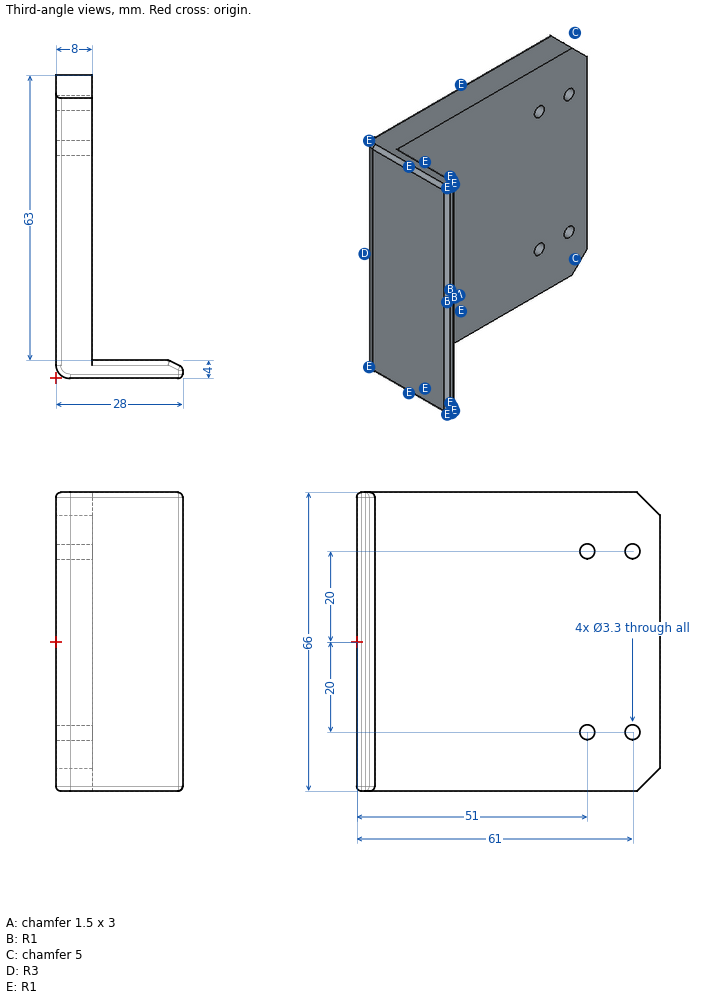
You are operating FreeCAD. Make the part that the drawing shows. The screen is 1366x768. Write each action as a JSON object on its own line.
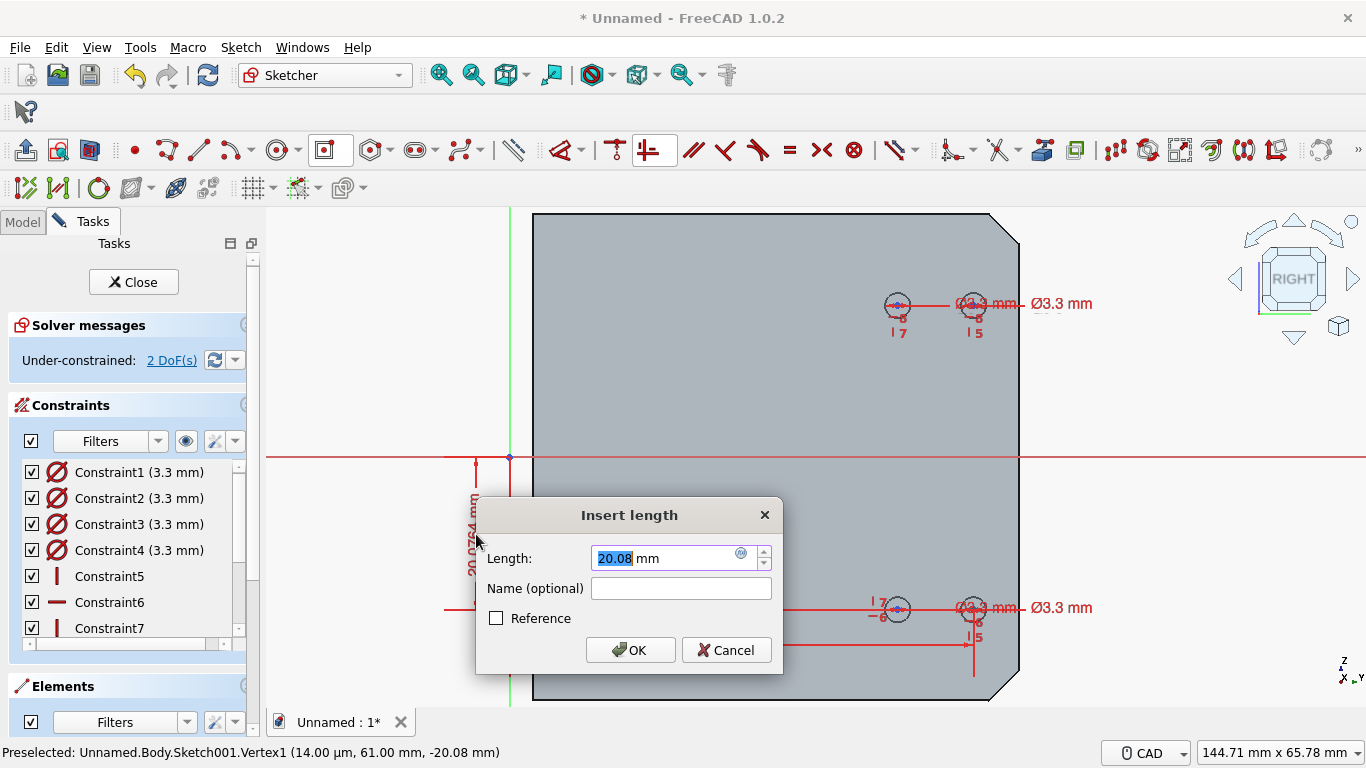
{"action": "type", "text": "20"}
{"action": "key", "text": "Return"}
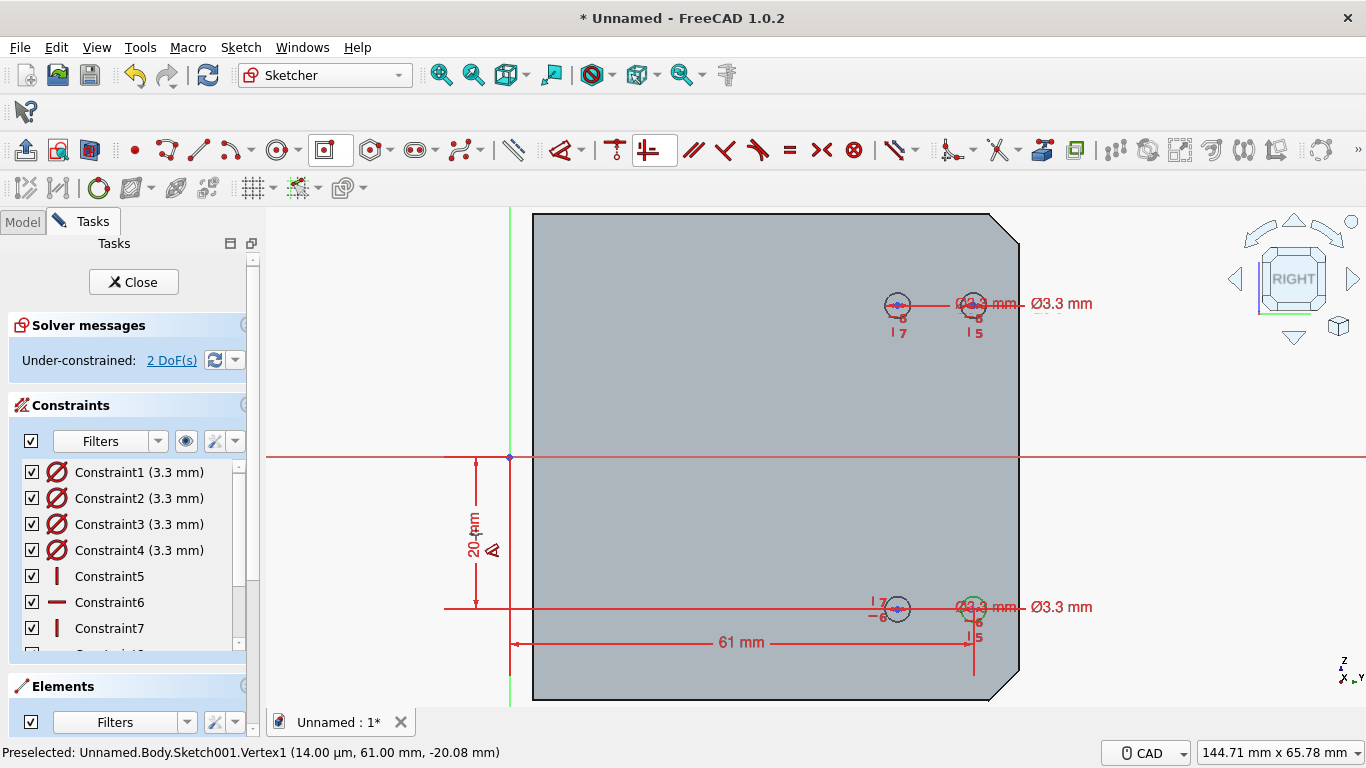
{"action": "left_click", "coordinate": [974, 306]}
{"action": "left_click", "coordinate": [476, 381]}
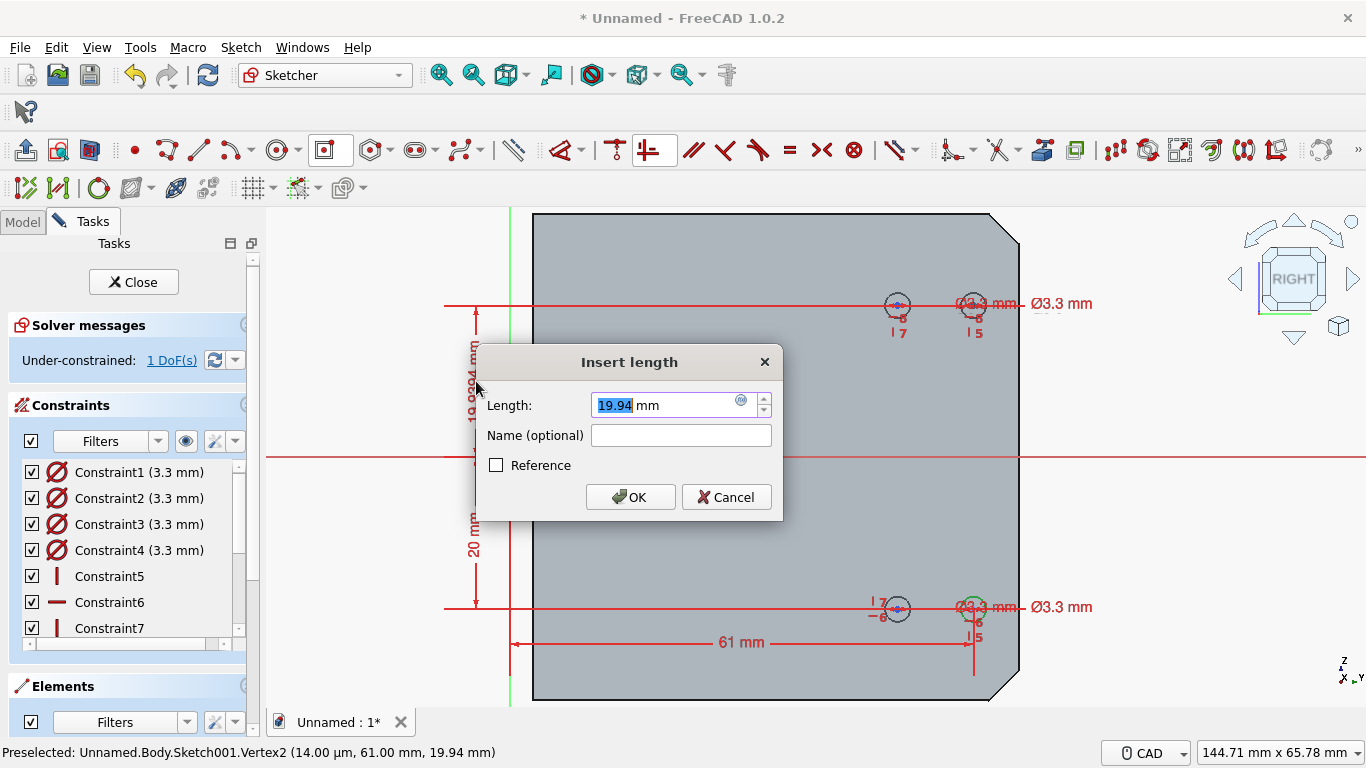
{"action": "type", "text": "20"}
{"action": "key", "text": "Return"}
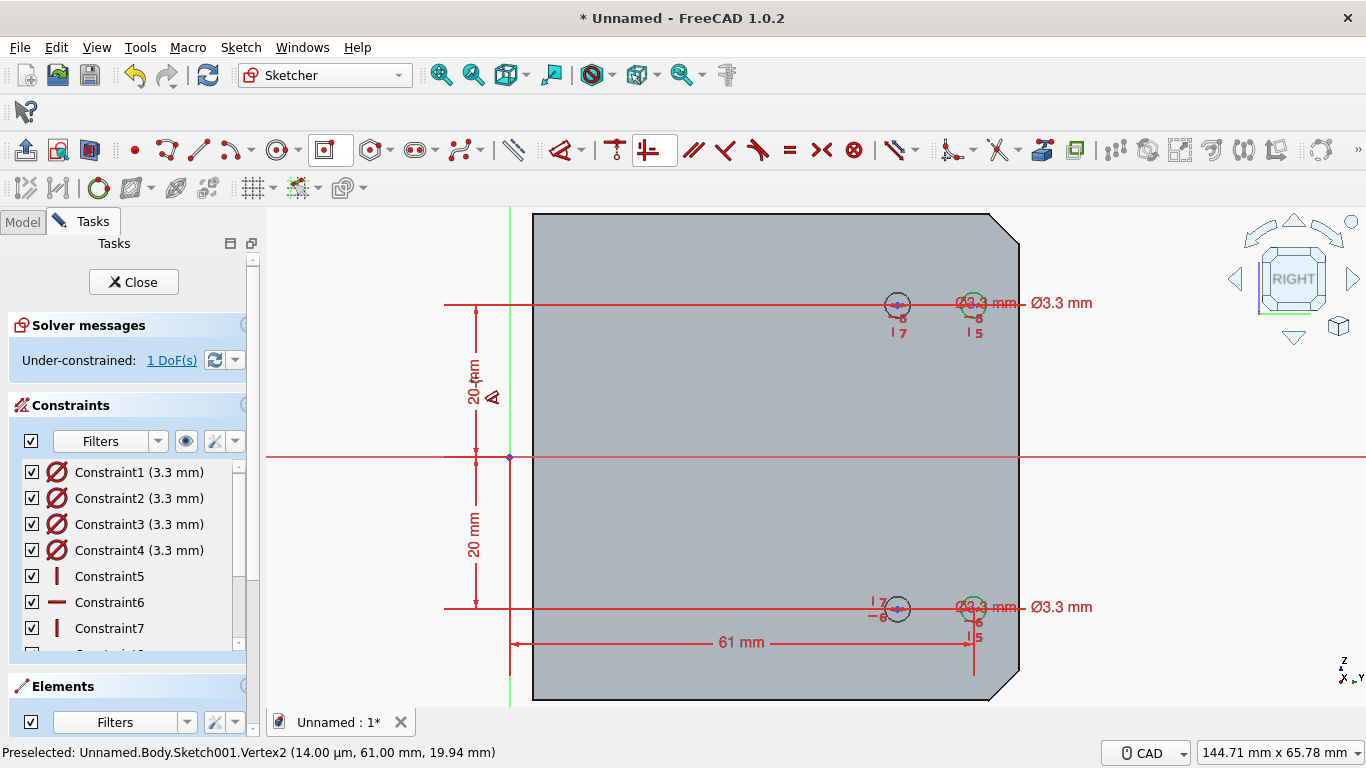
{"action": "left_click", "coordinate": [898, 609]}
{"action": "left_click", "coordinate": [615, 643]}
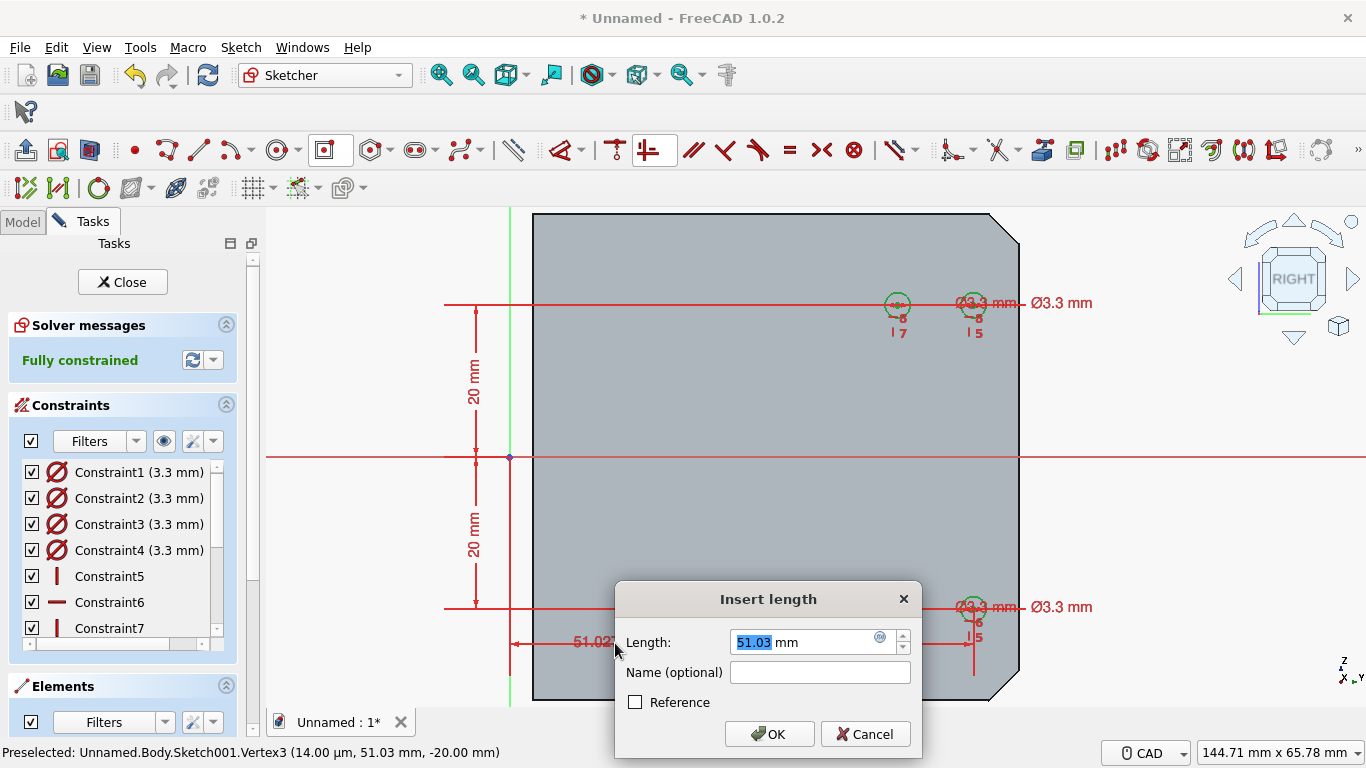
{"action": "type", "text": "51"}
{"action": "key", "text": "Return"}
{"action": "key", "text": "Escape"}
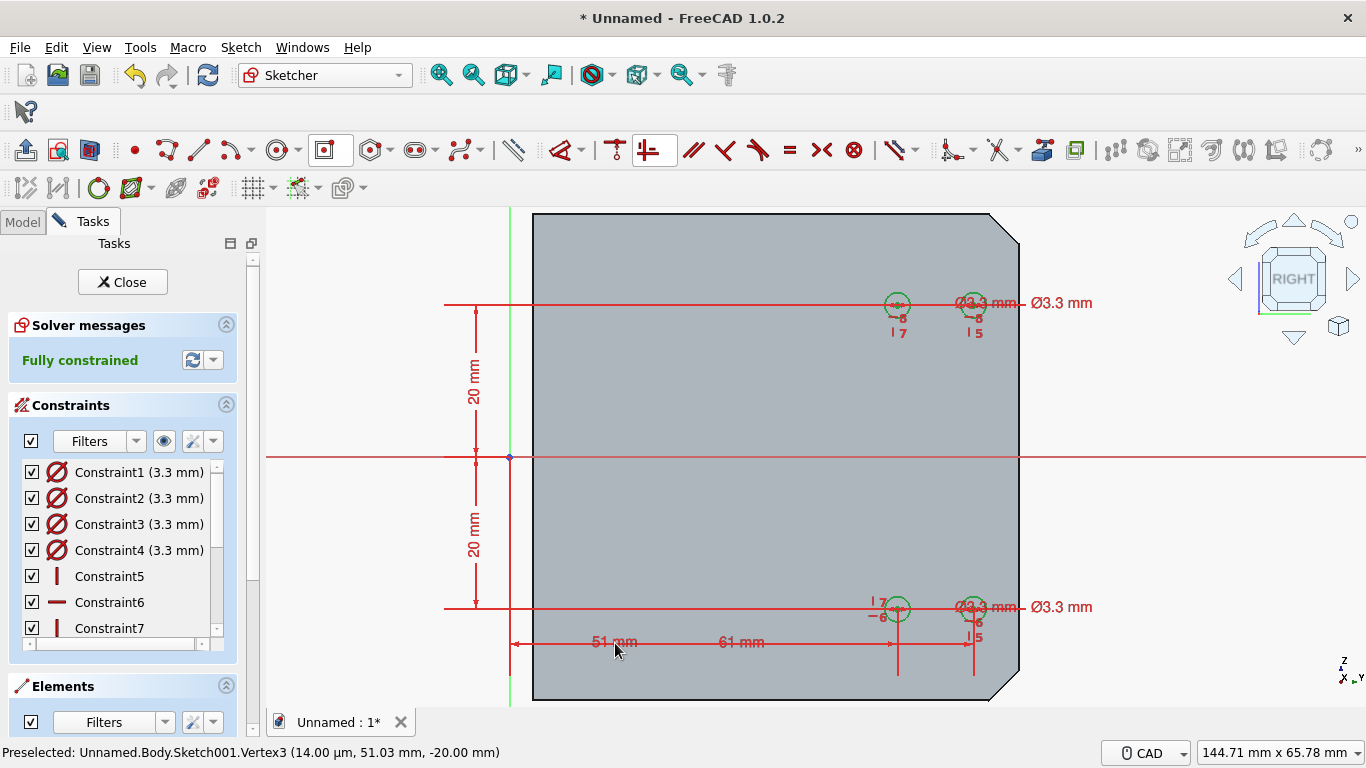
{"action": "left_click", "coordinate": [123, 282]}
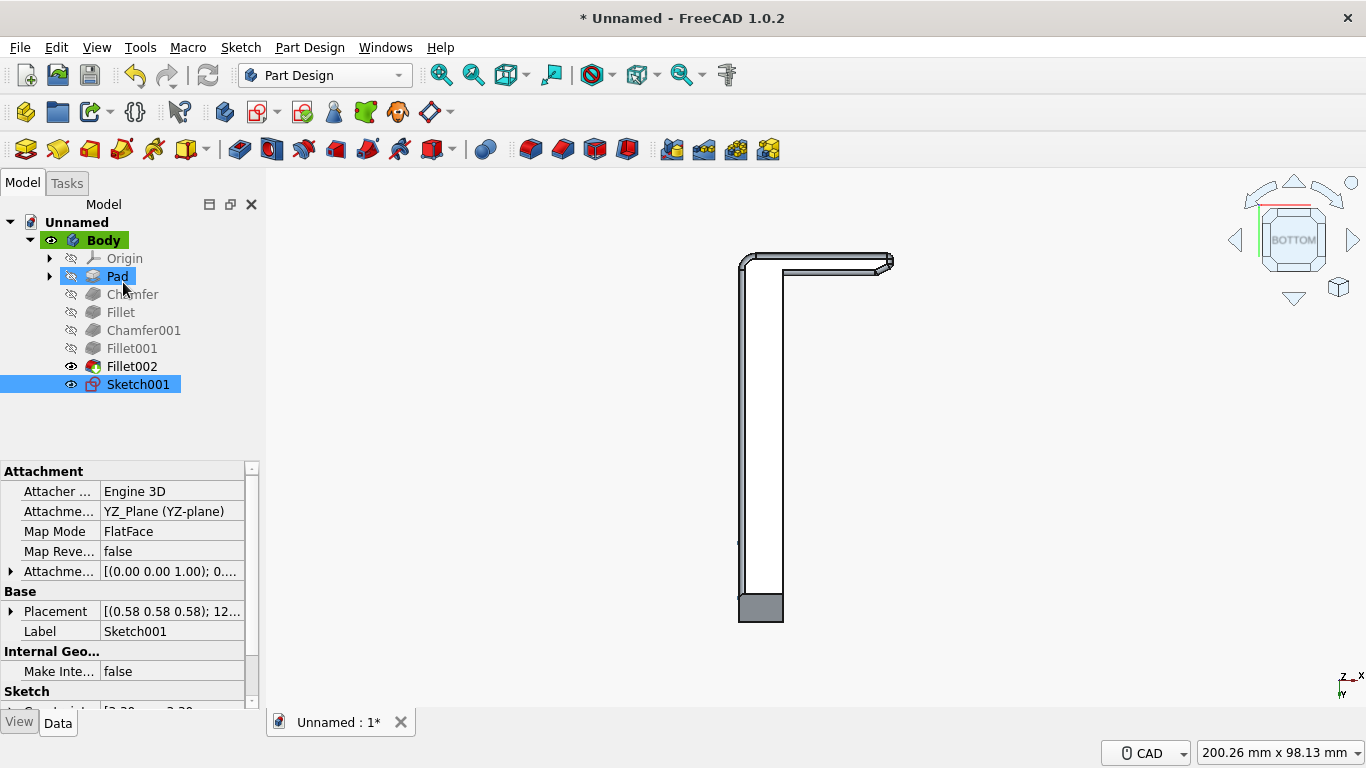
{"action": "left_click", "coordinate": [272, 150]}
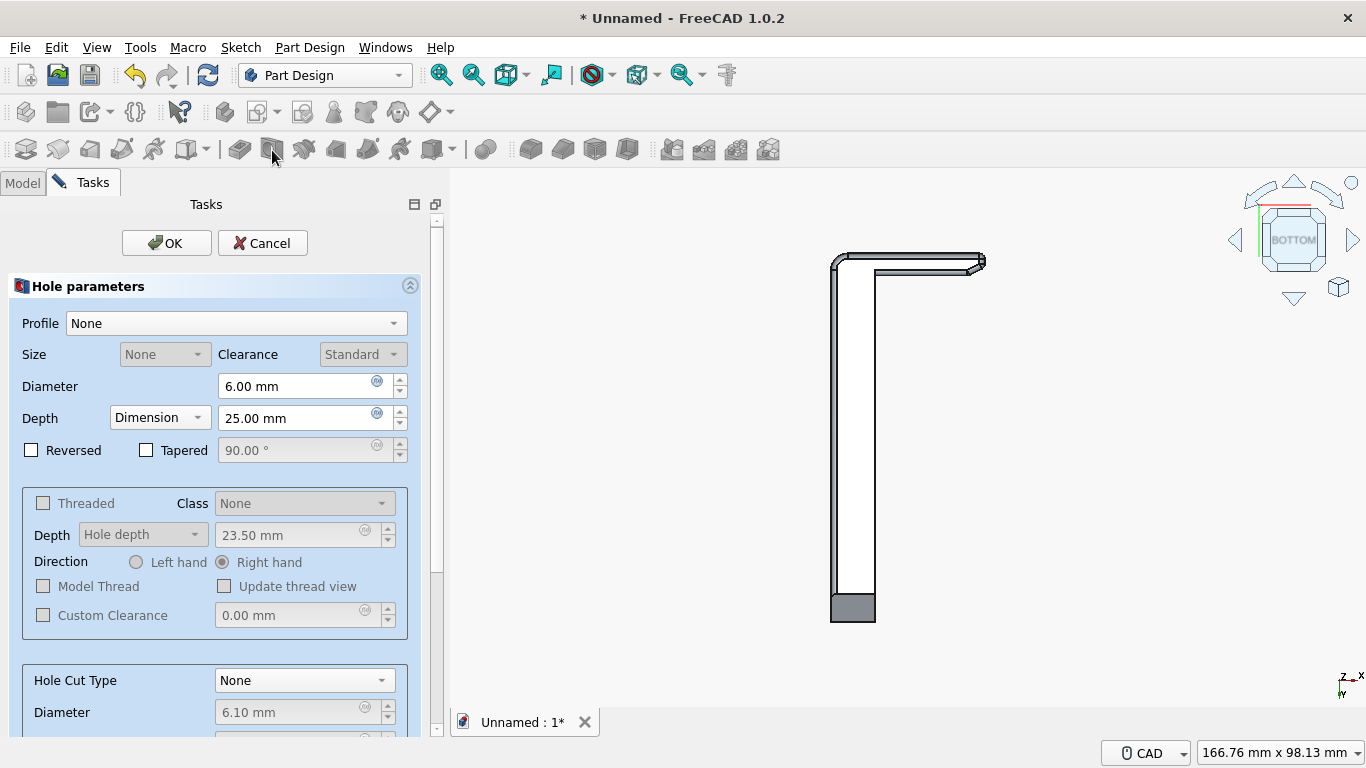
{"action": "triple_click", "coordinate": [305, 386]}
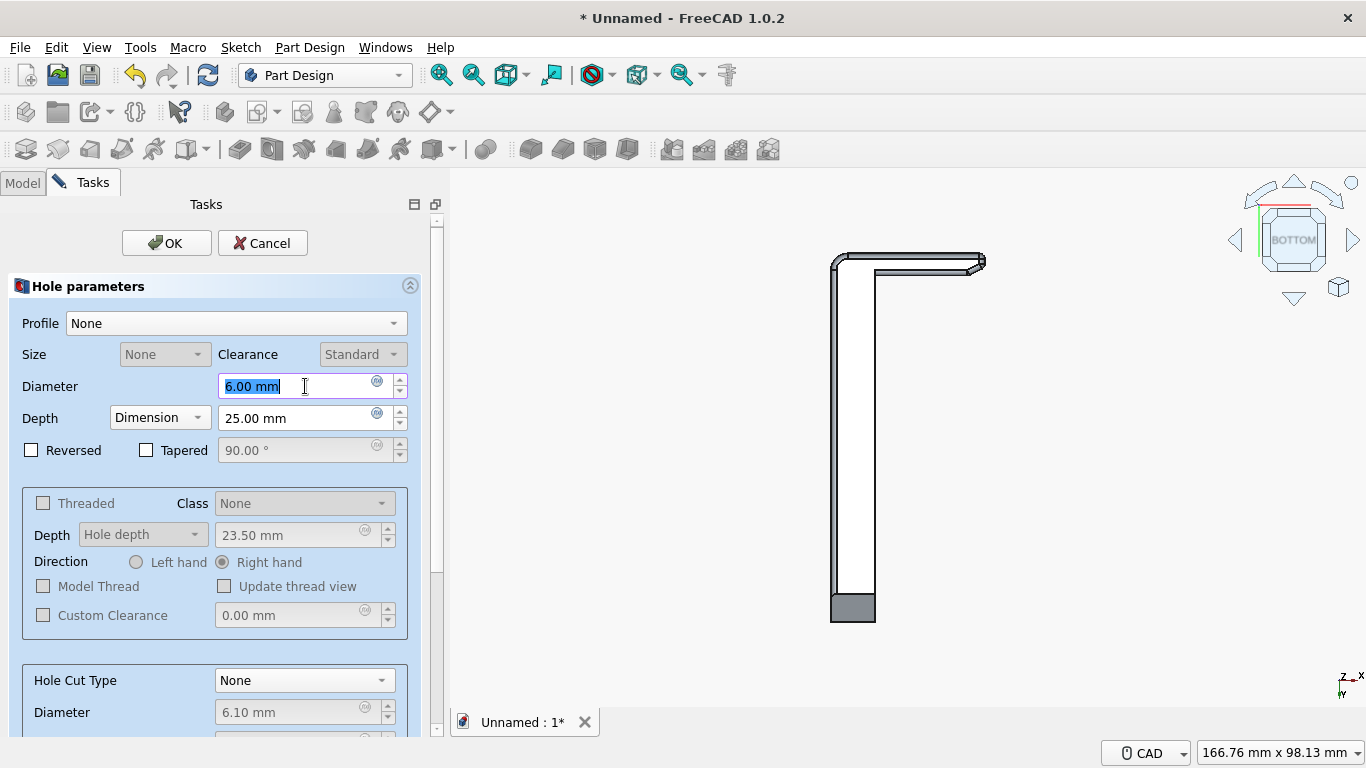
{"action": "type", "text": "3.3"}
{"action": "key", "text": "Tab"}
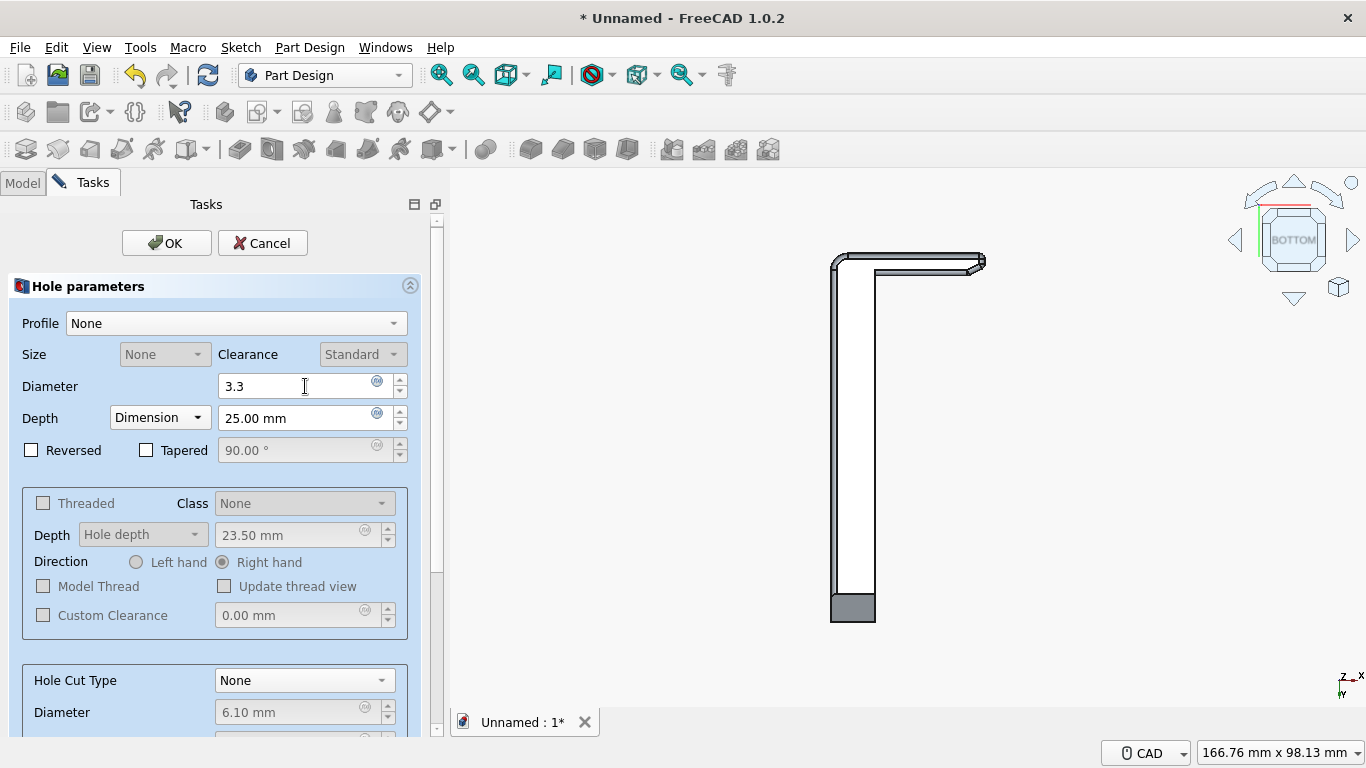
{"action": "left_click", "coordinate": [161, 418]}